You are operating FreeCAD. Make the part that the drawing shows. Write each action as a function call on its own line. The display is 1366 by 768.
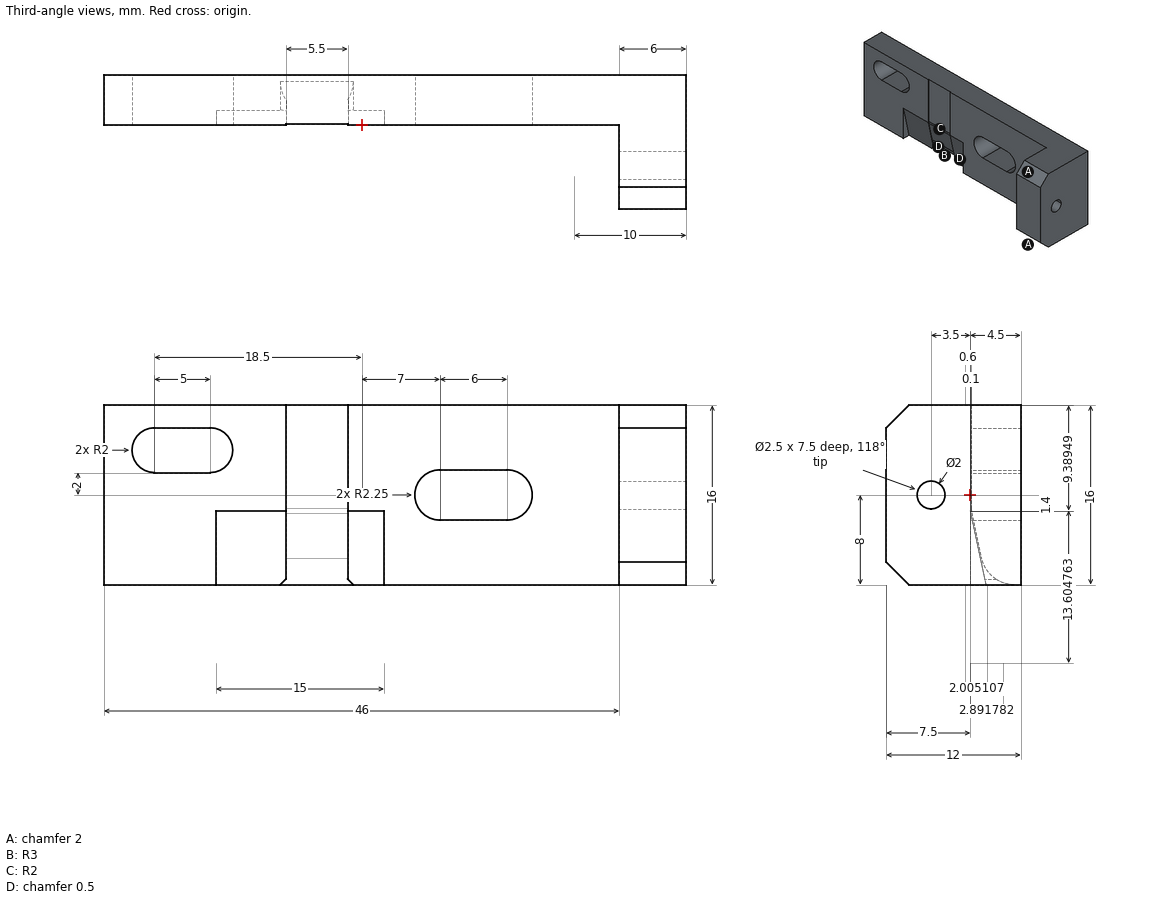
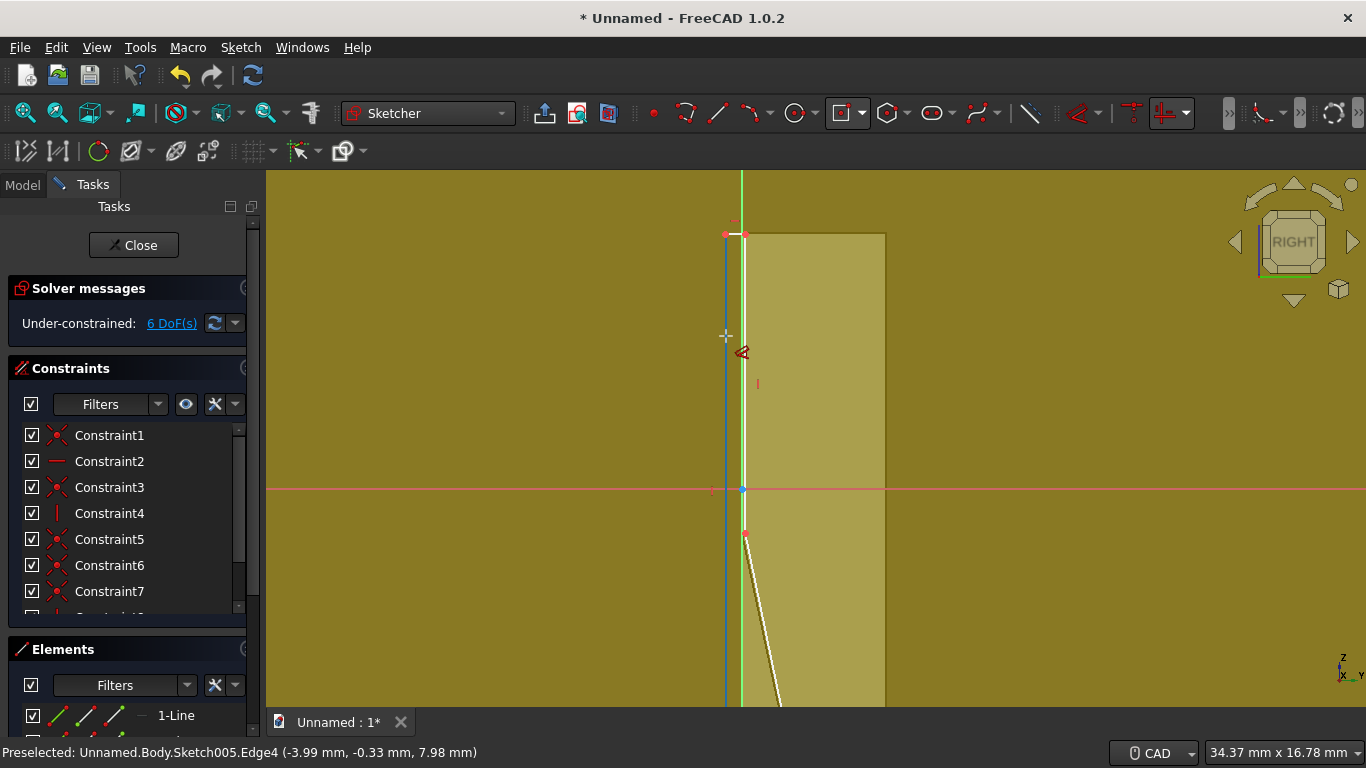
click(726, 337)
click(692, 457)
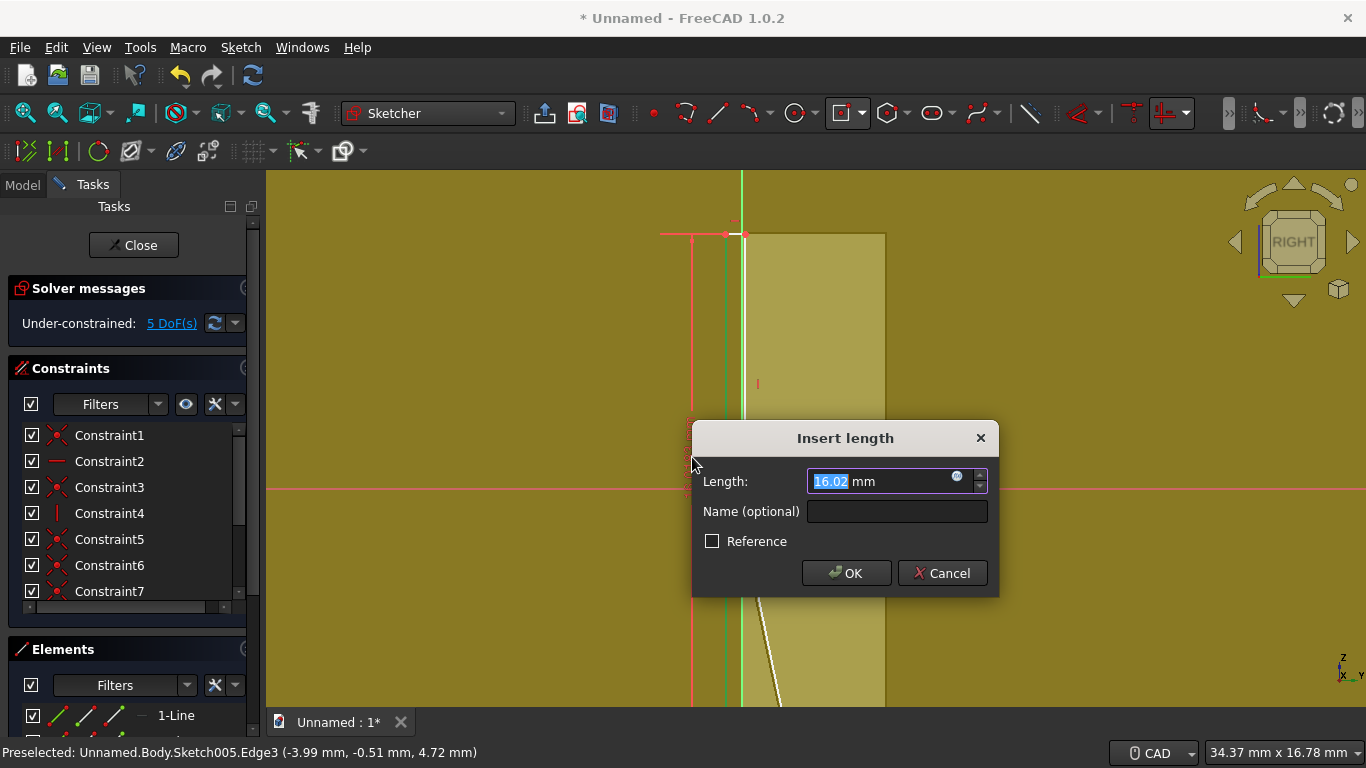
text(16)
key(Return)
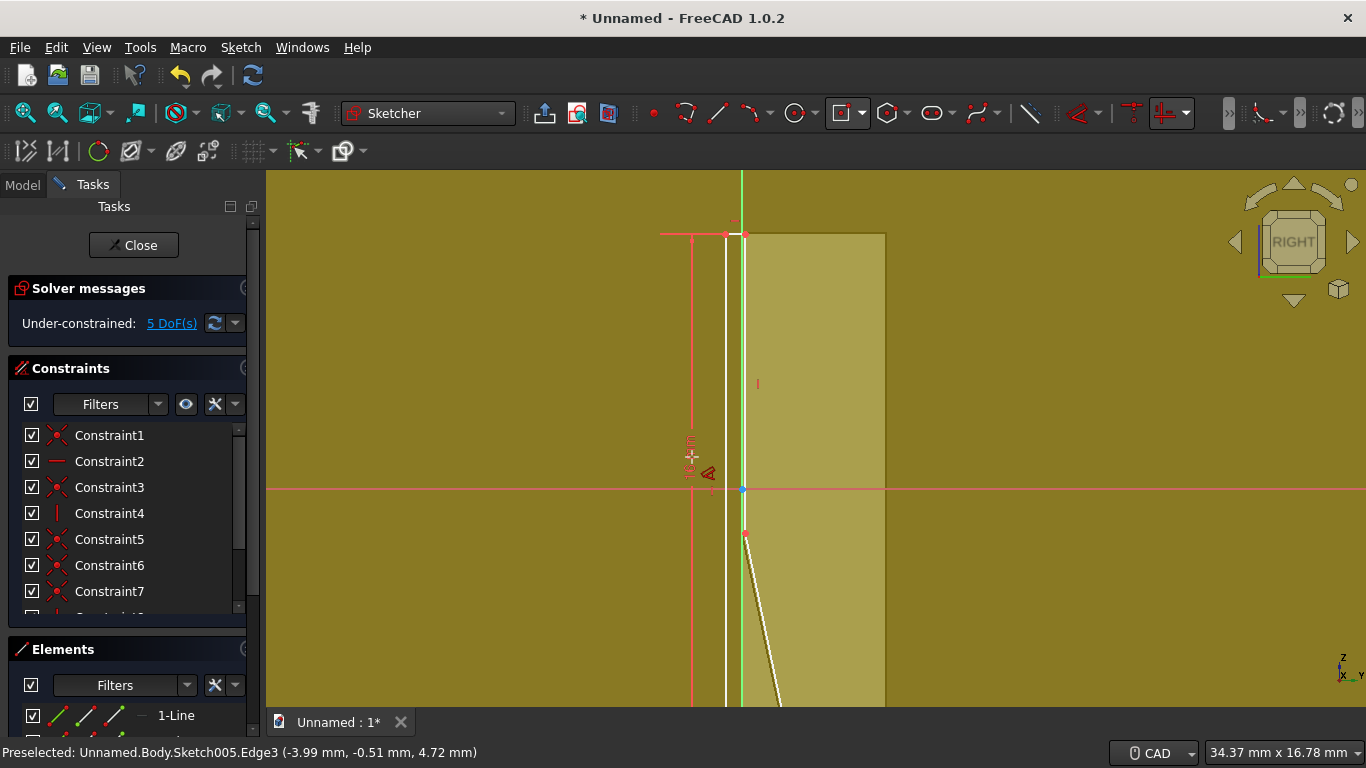
scroll(726, 336, down, 2)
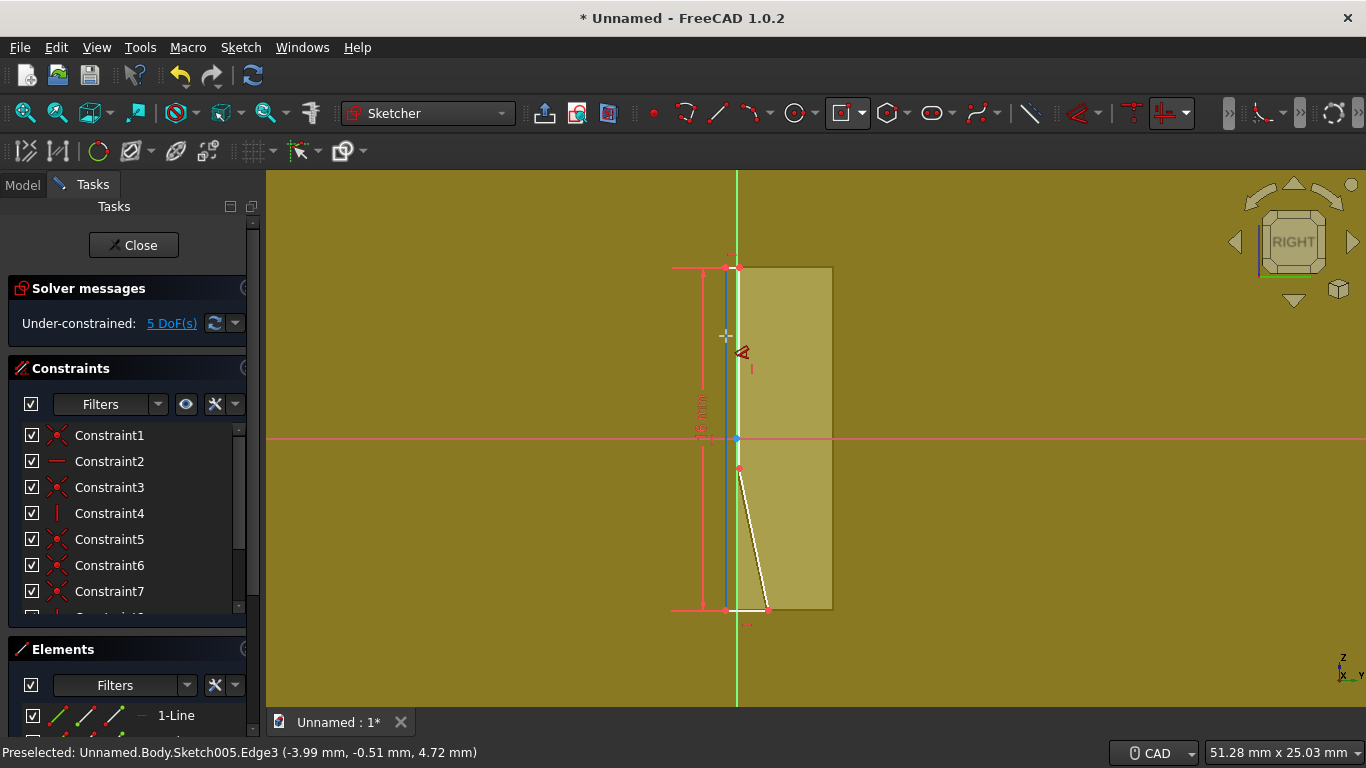
click(769, 611)
click(803, 525)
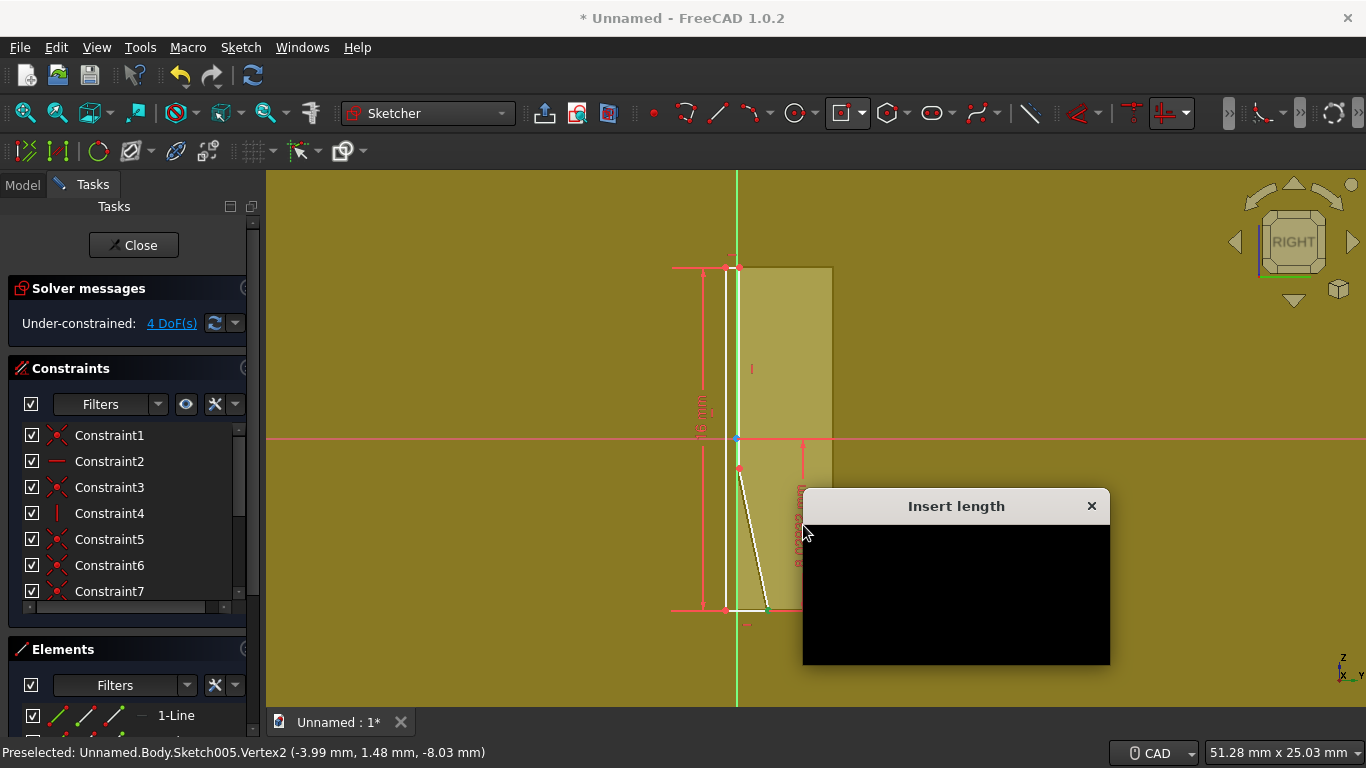
text(8)
key(Return)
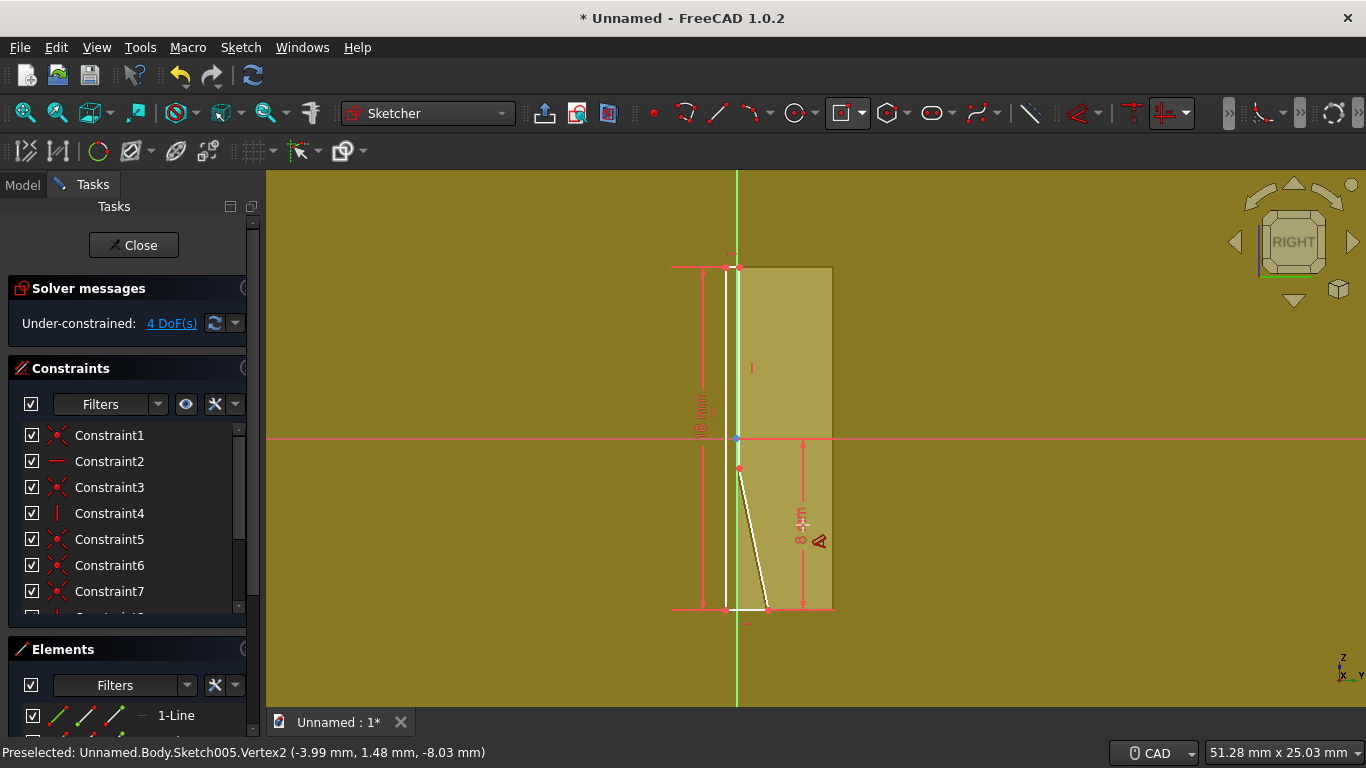
scroll(734, 267, up, 6)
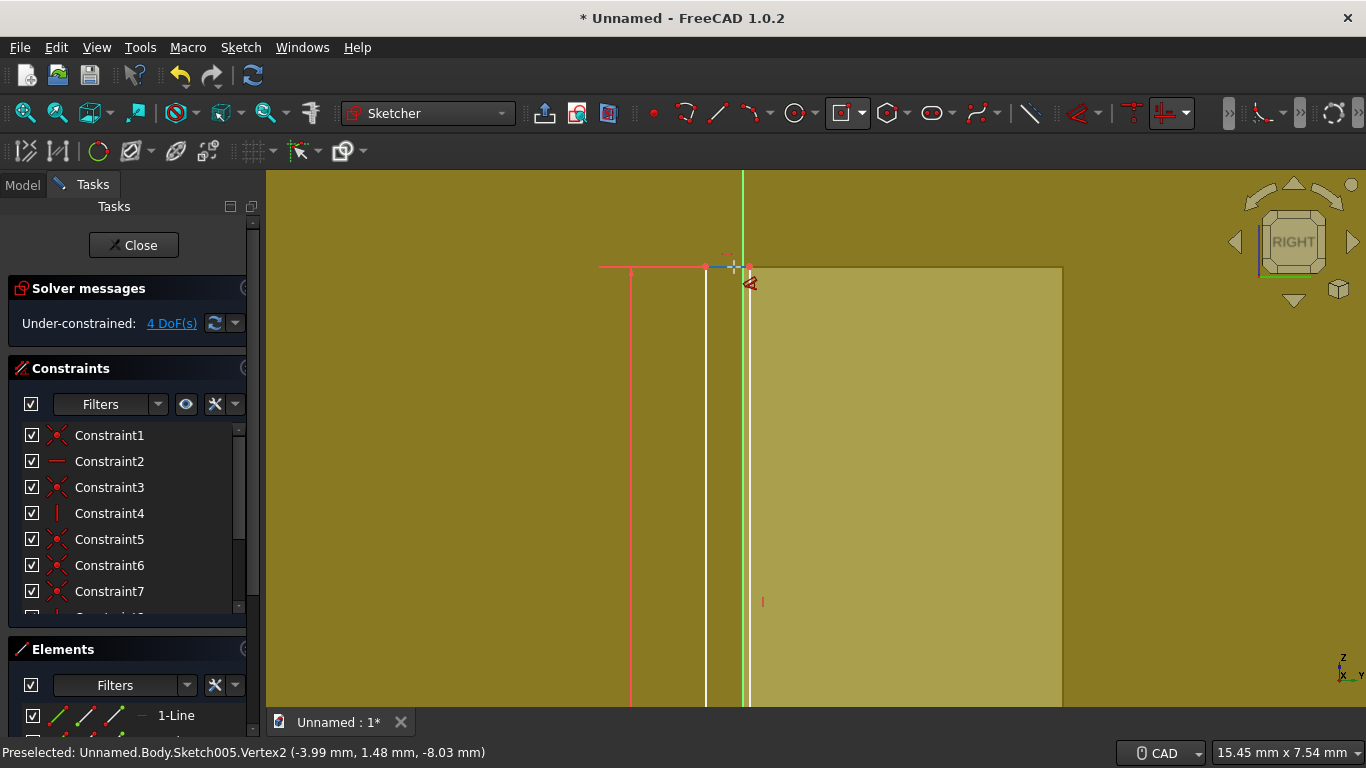
click(732, 267)
click(728, 233)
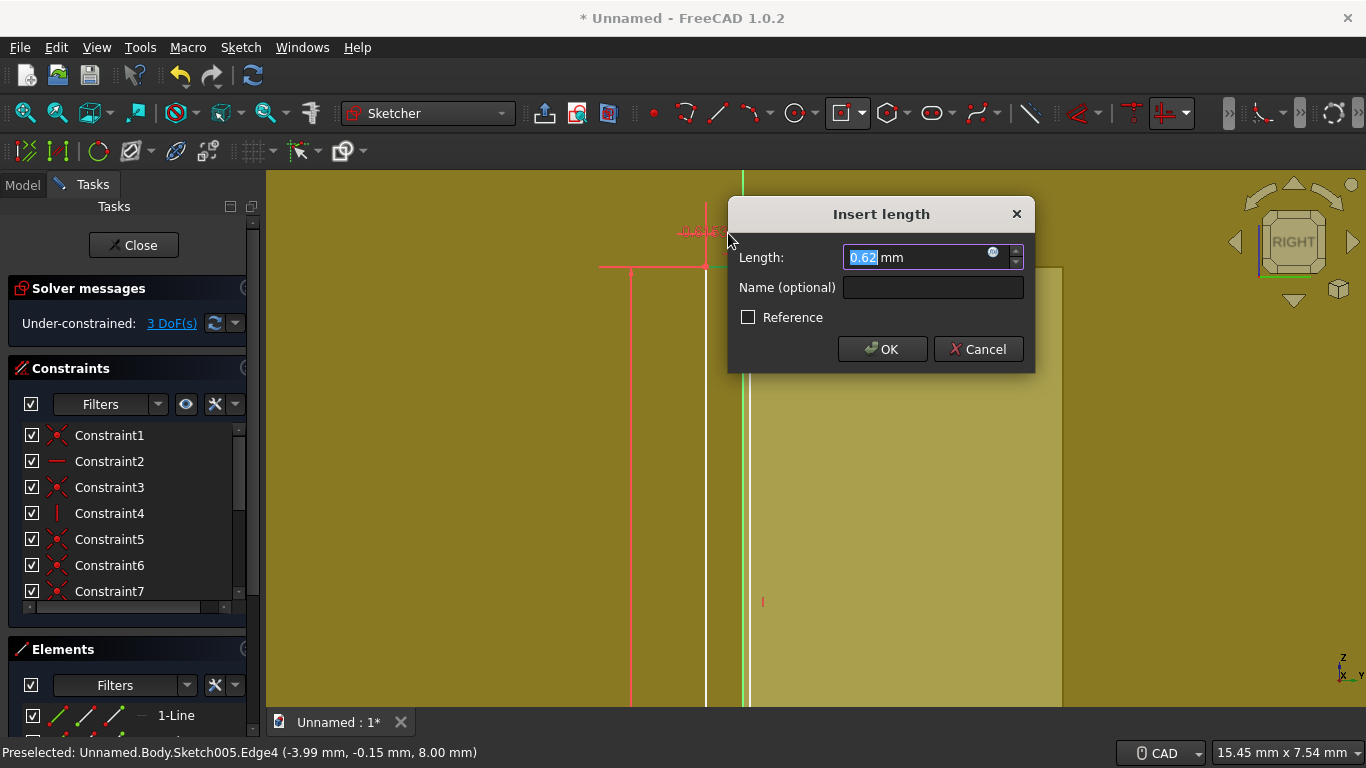
text(0.6)
key(Return)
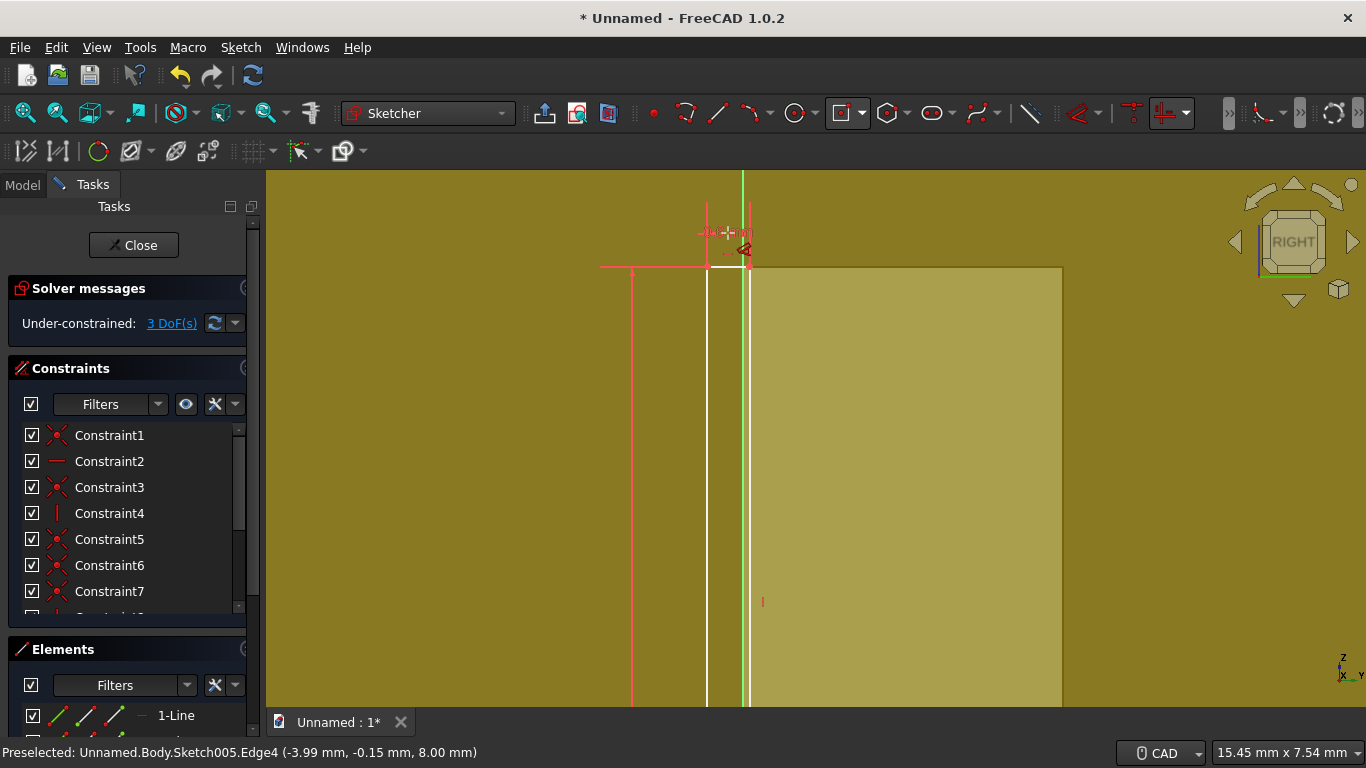
scroll(734, 267, down, 6)